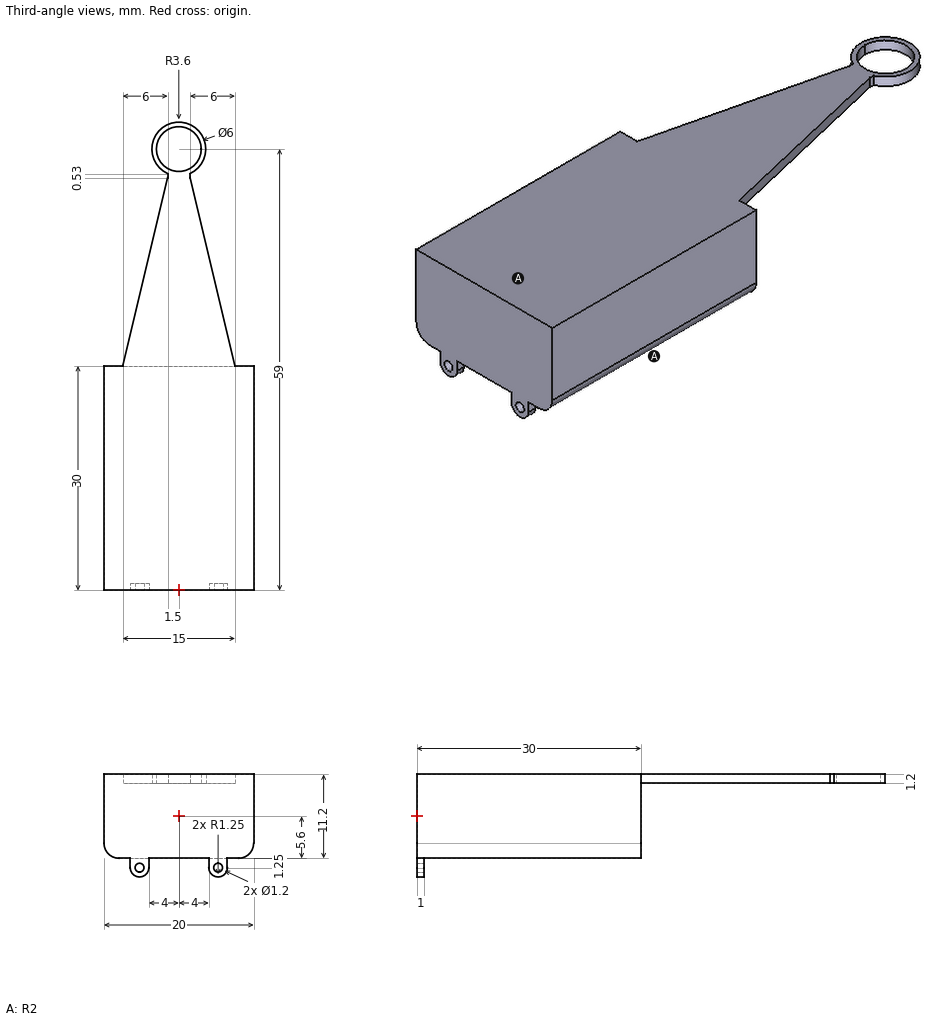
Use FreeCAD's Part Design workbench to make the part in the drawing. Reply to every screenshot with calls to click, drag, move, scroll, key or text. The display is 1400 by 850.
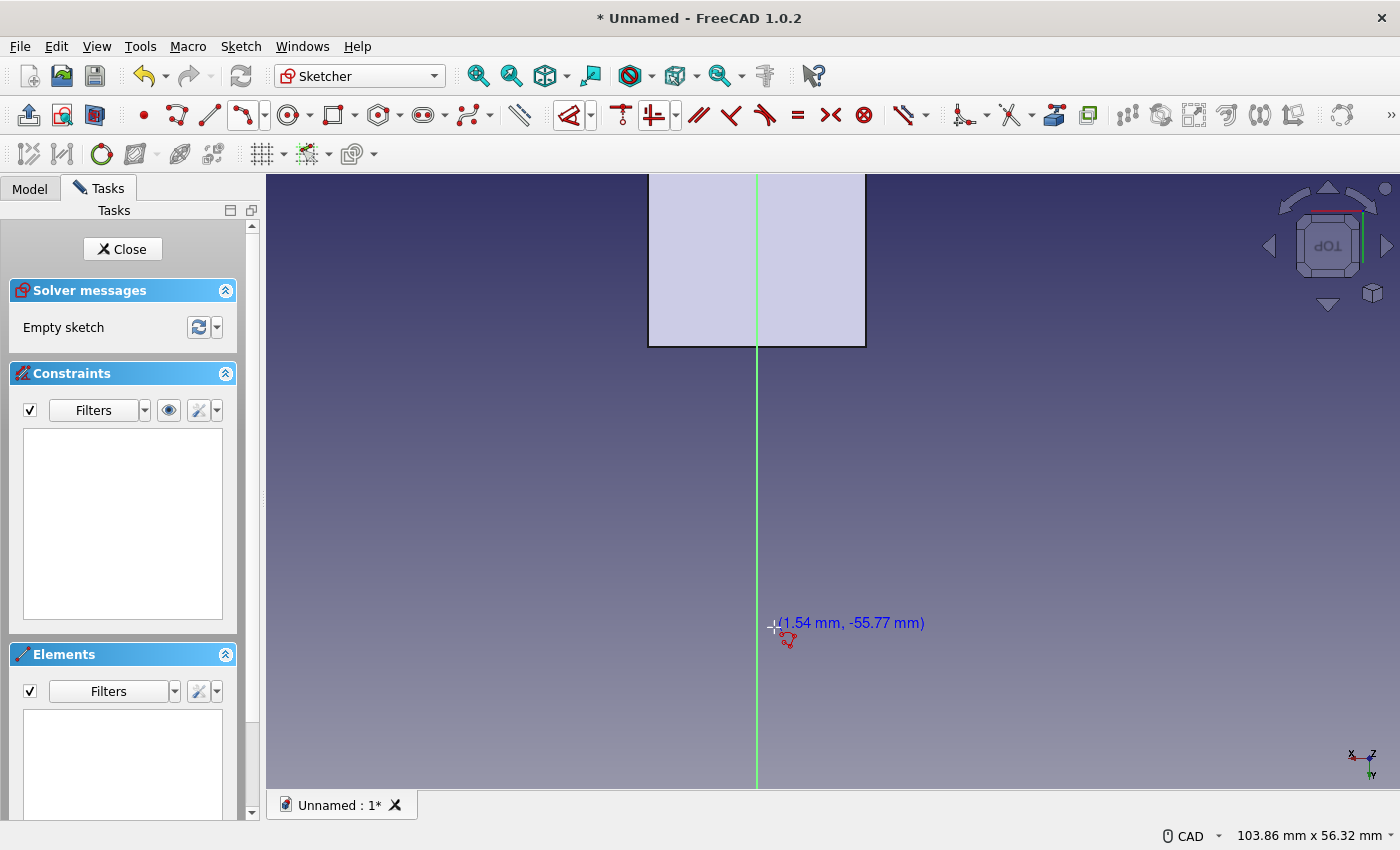
scroll(774, 622, up, 6)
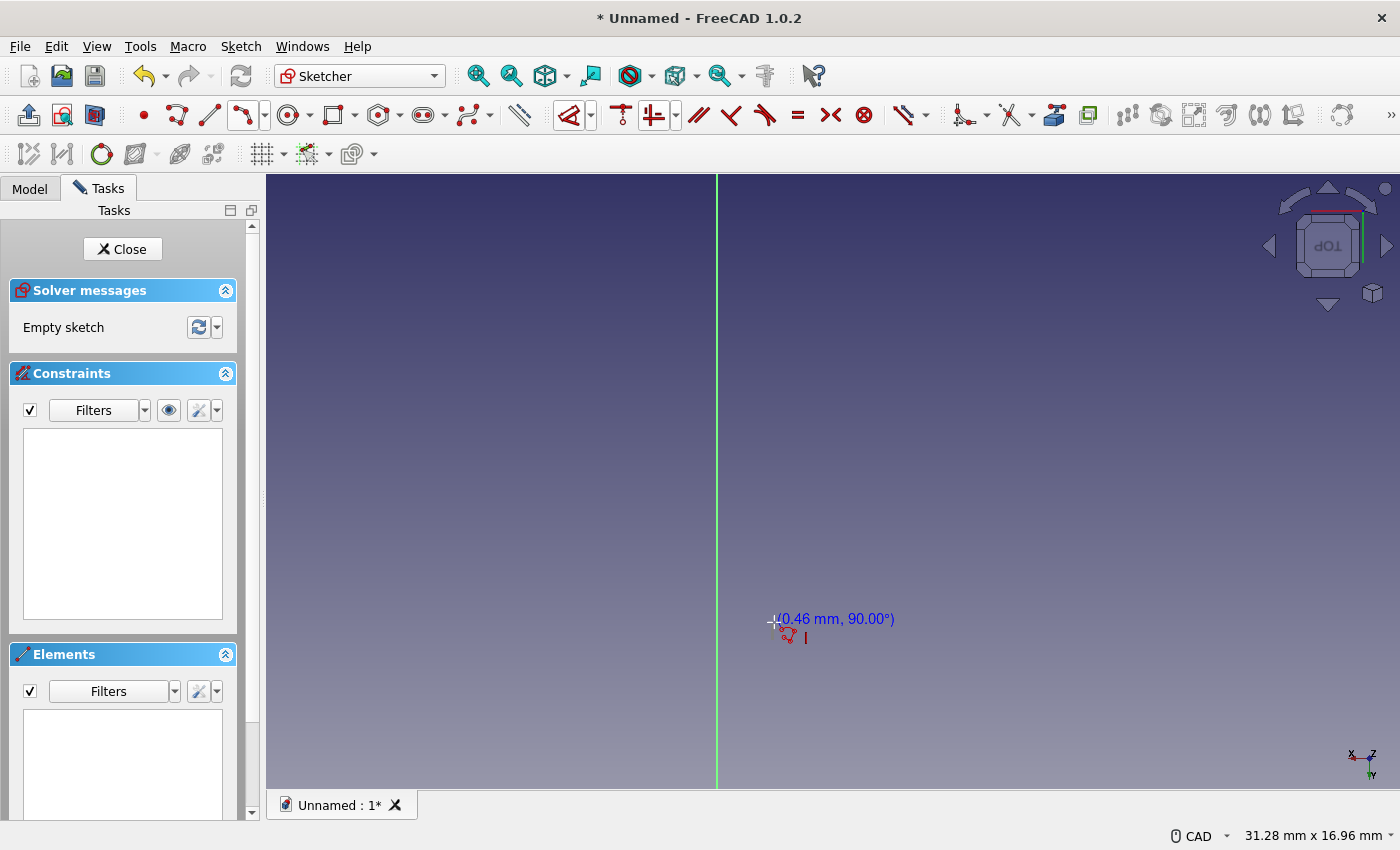
click(773, 619)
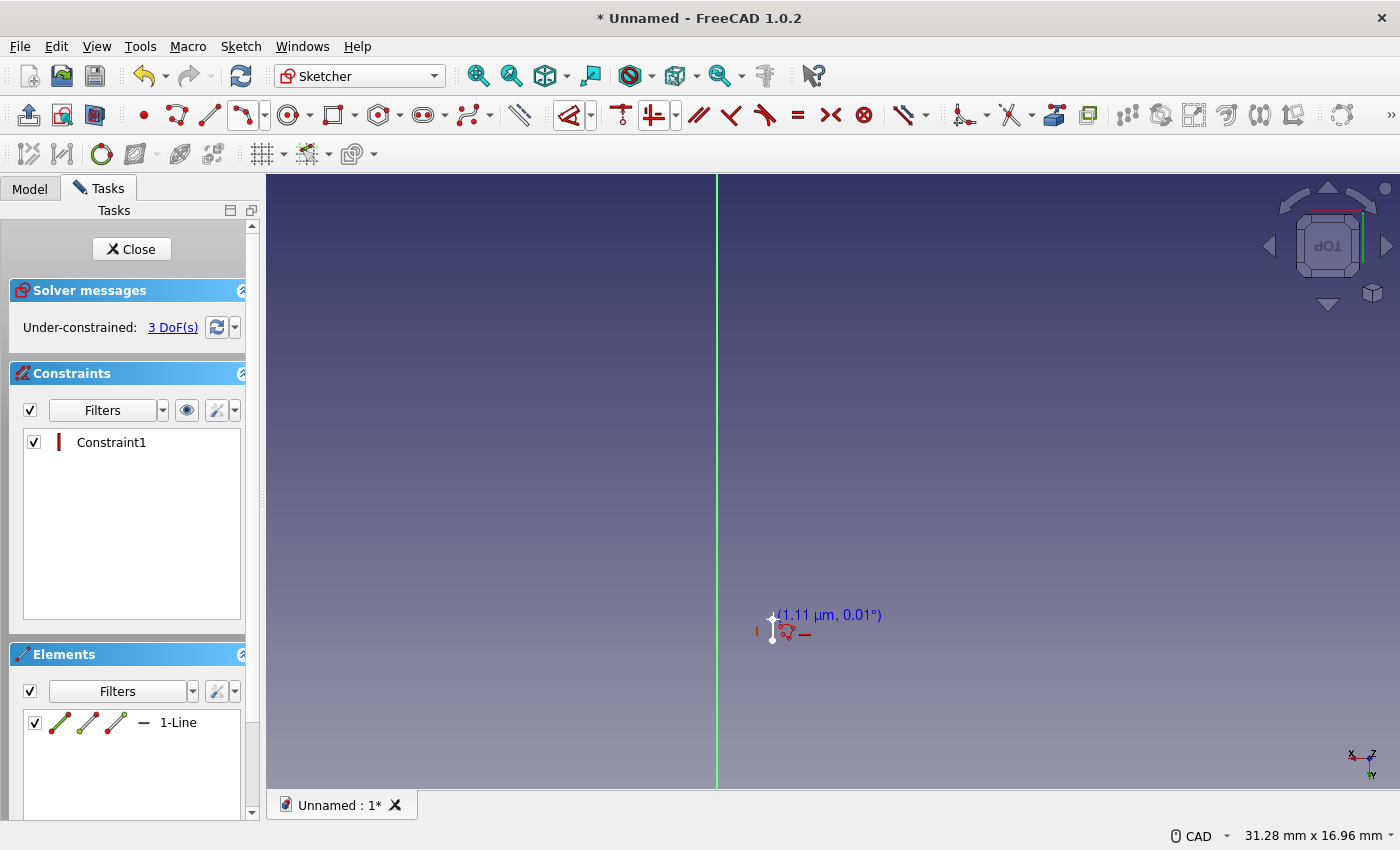
scroll(774, 626, down, 9)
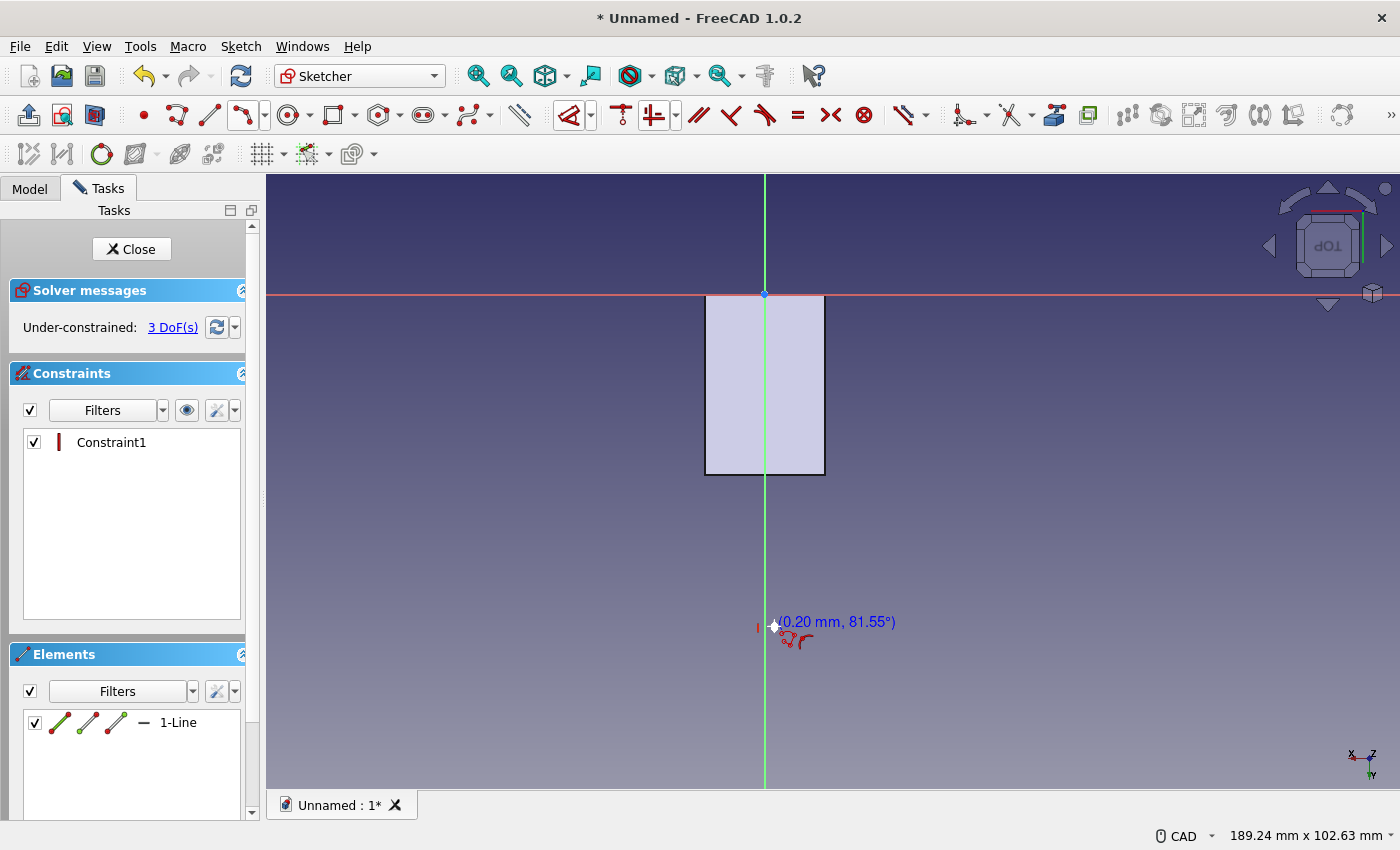
click(810, 475)
click(720, 475)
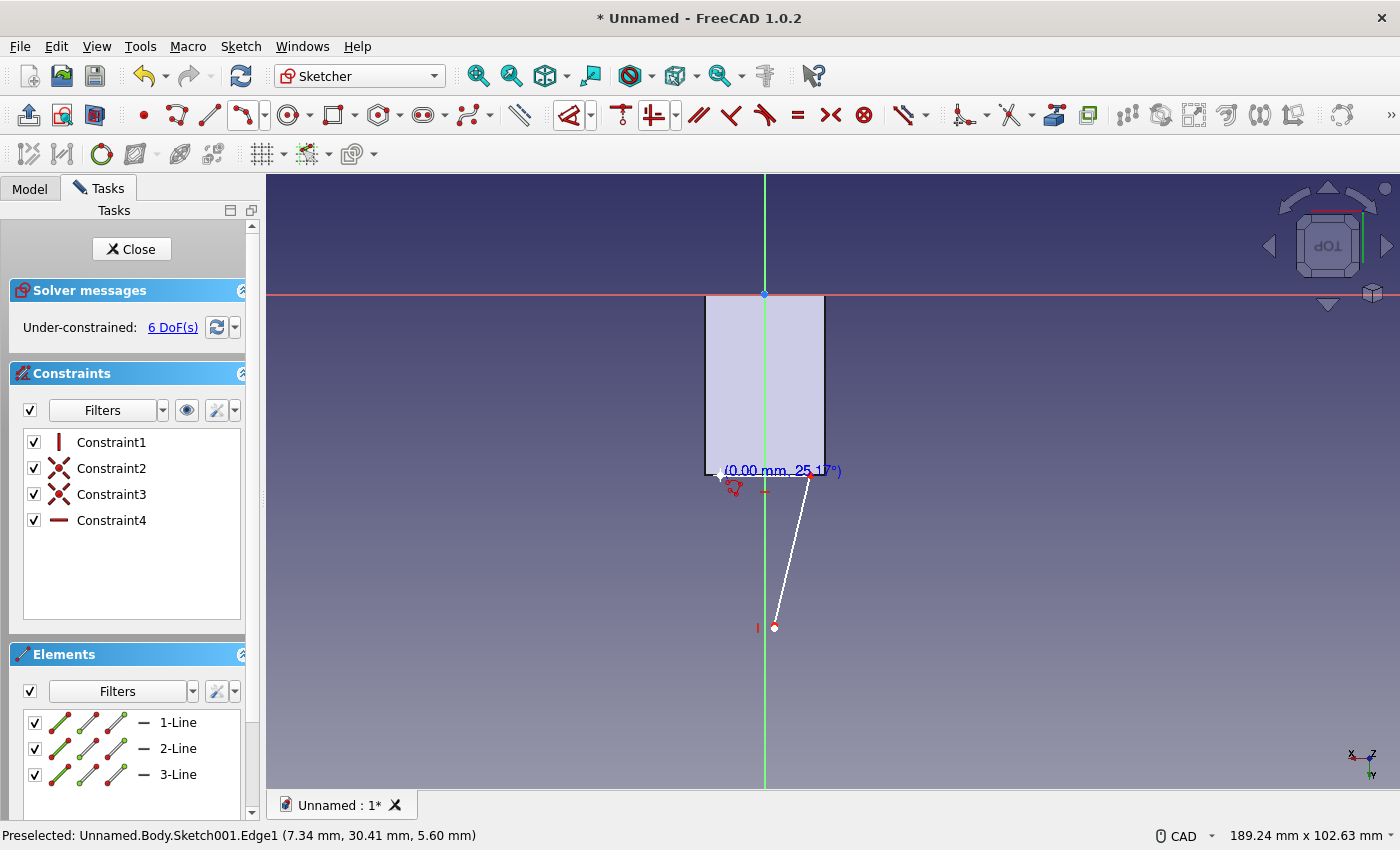
scroll(756, 626, up, 3)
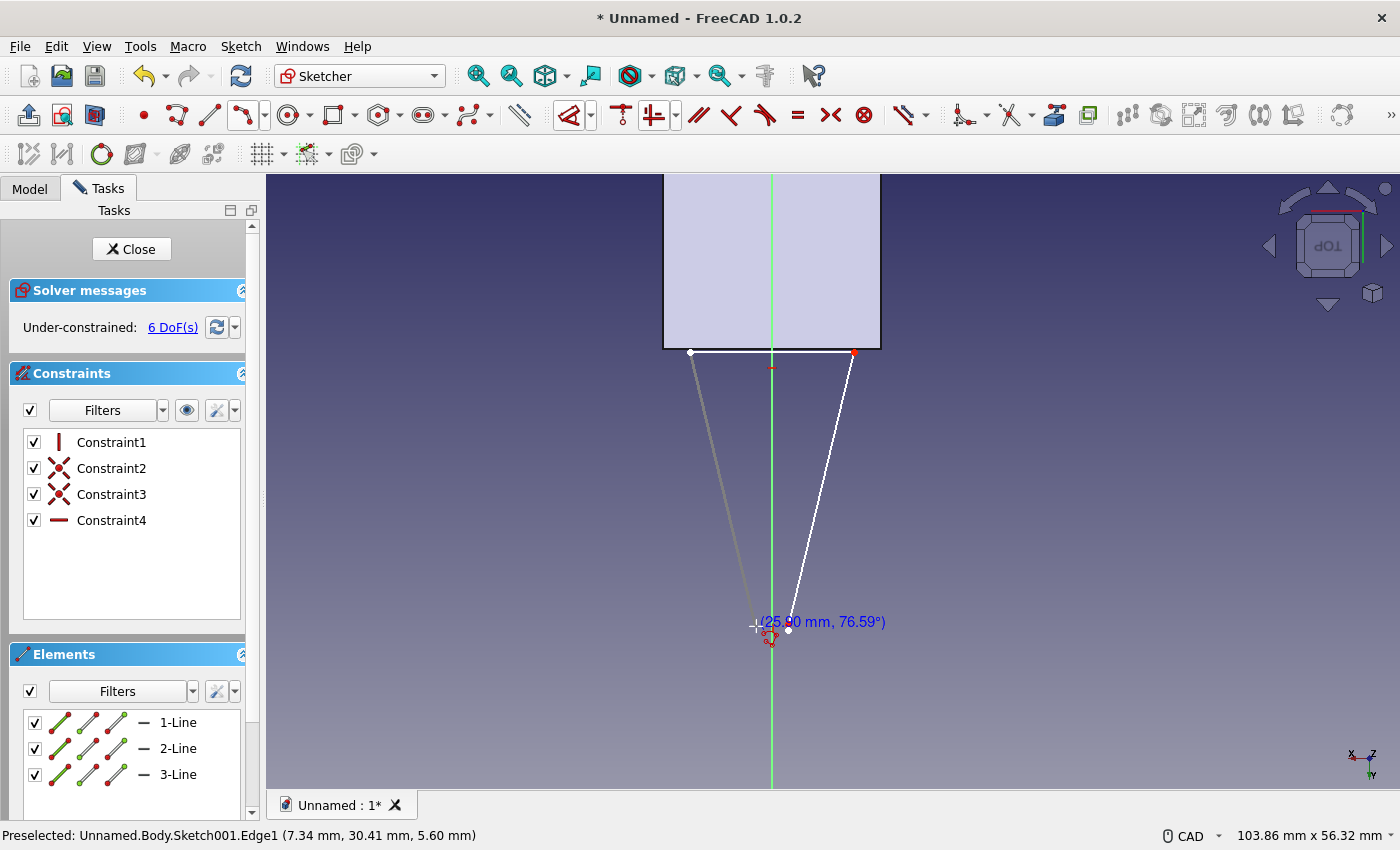
click(756, 625)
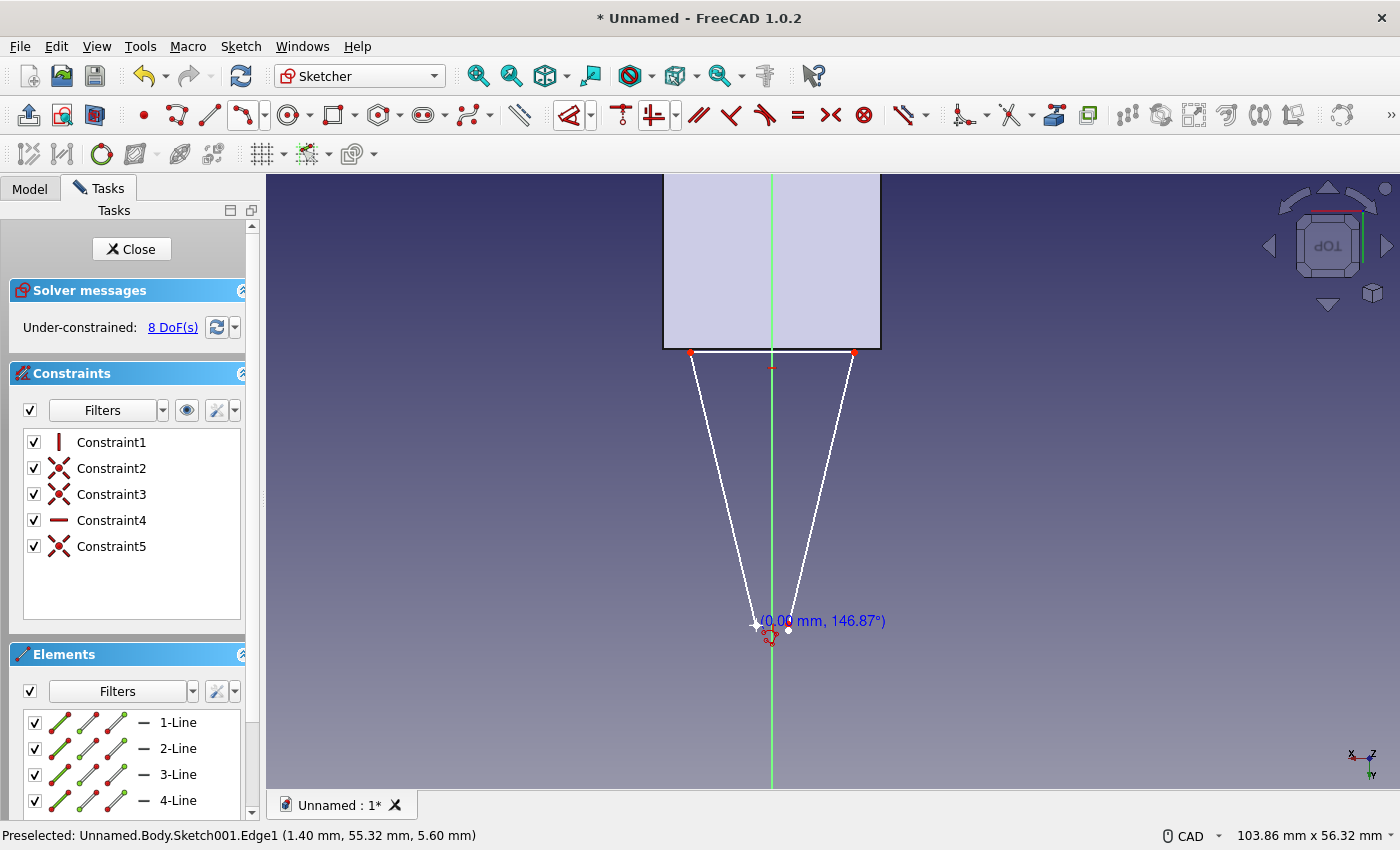
scroll(756, 630, up, 6)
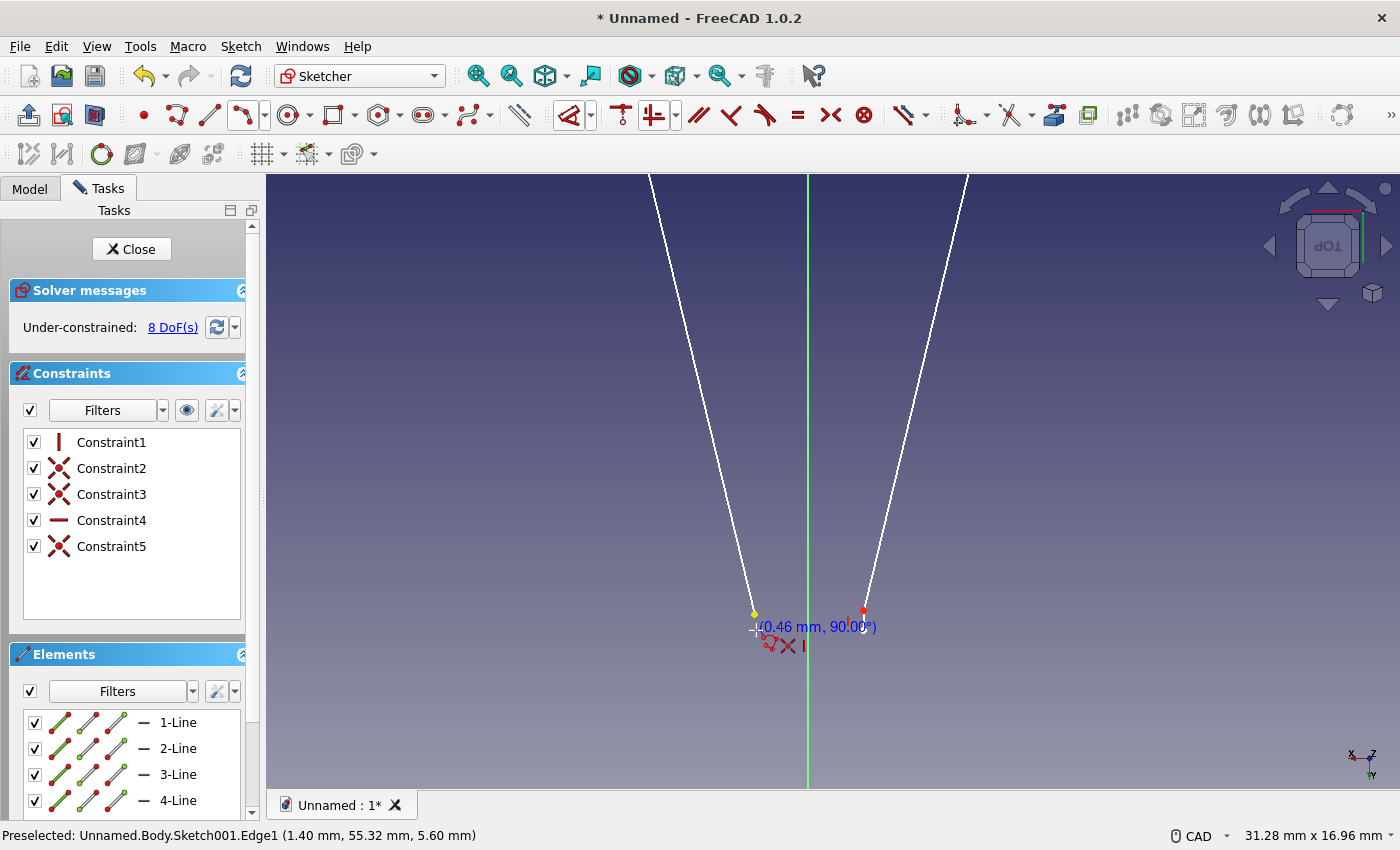
click(755, 629)
right_click(755, 629)